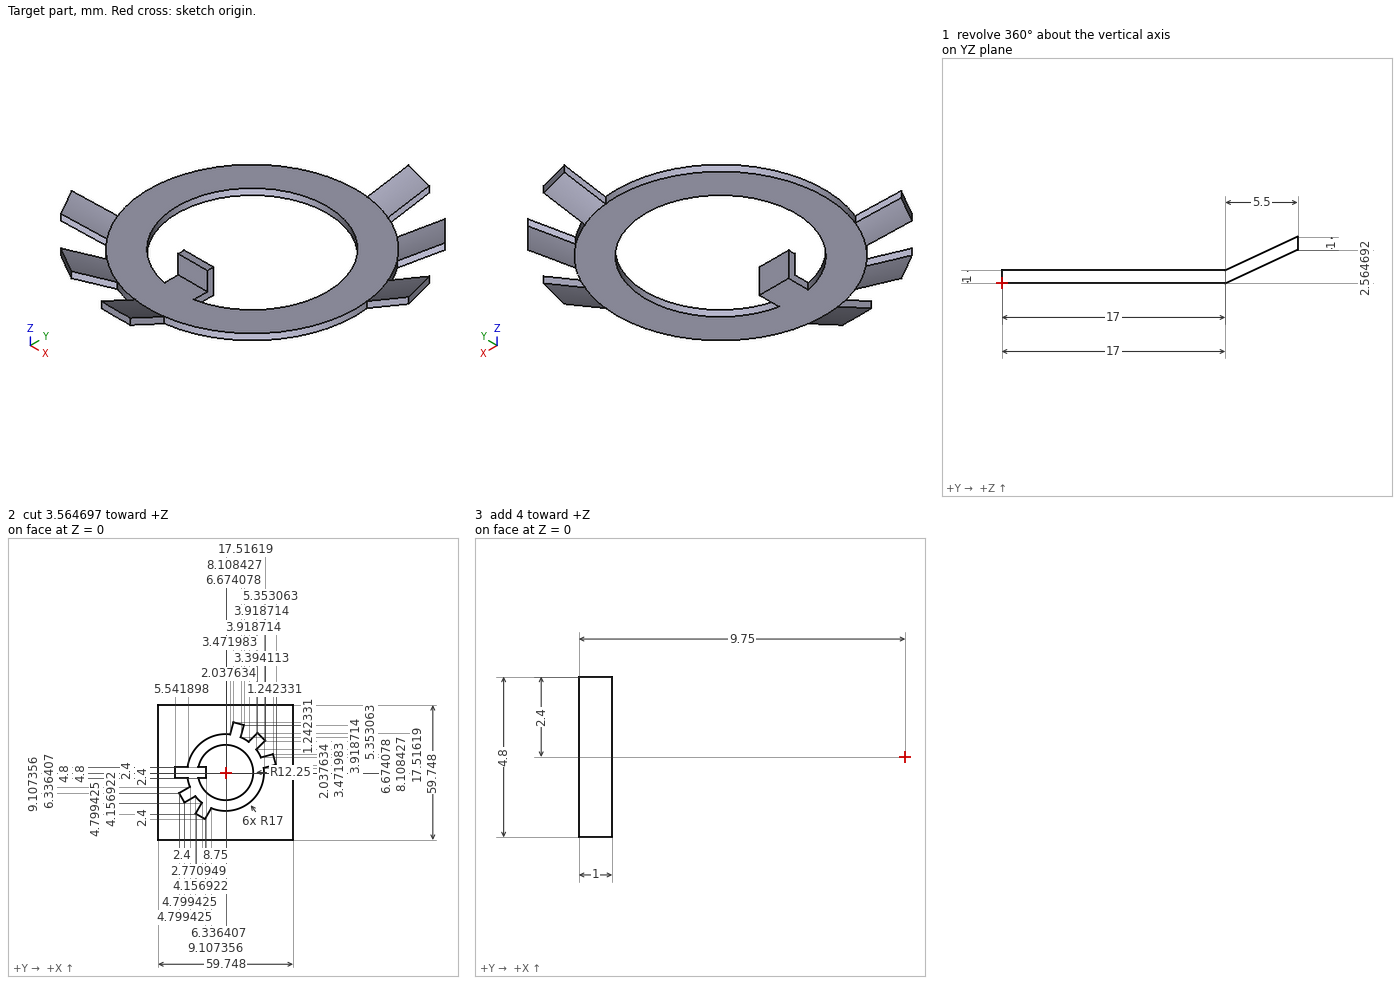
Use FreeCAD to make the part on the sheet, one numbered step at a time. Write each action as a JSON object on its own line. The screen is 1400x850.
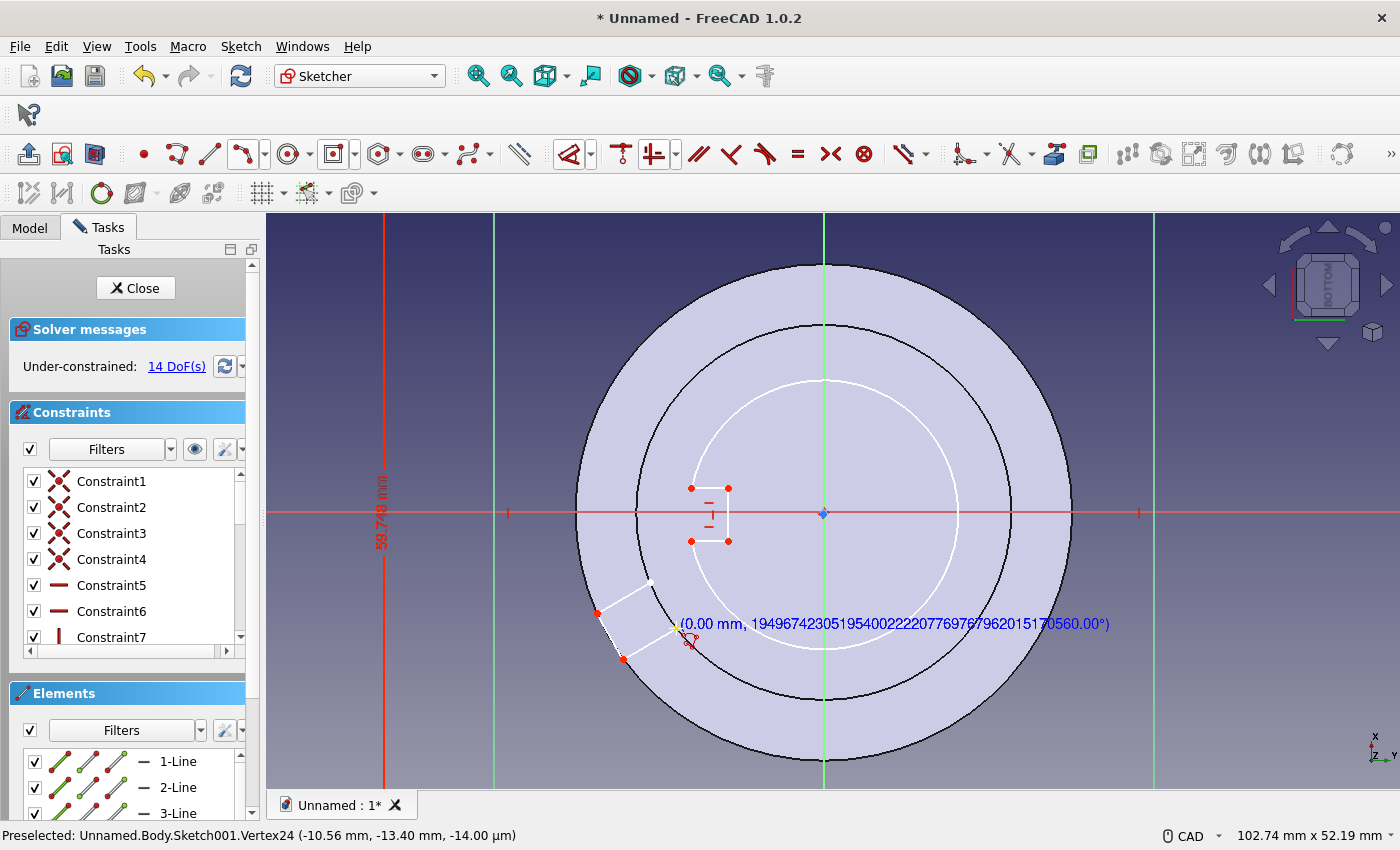
{"action": "left_click", "coordinate": [708, 660]}
{"action": "left_click", "coordinate": [677, 713]}
{"action": "left_click", "coordinate": [723, 740]}
{"action": "left_click", "coordinate": [754, 687]}
{"action": "right_click", "coordinate": [754, 687]}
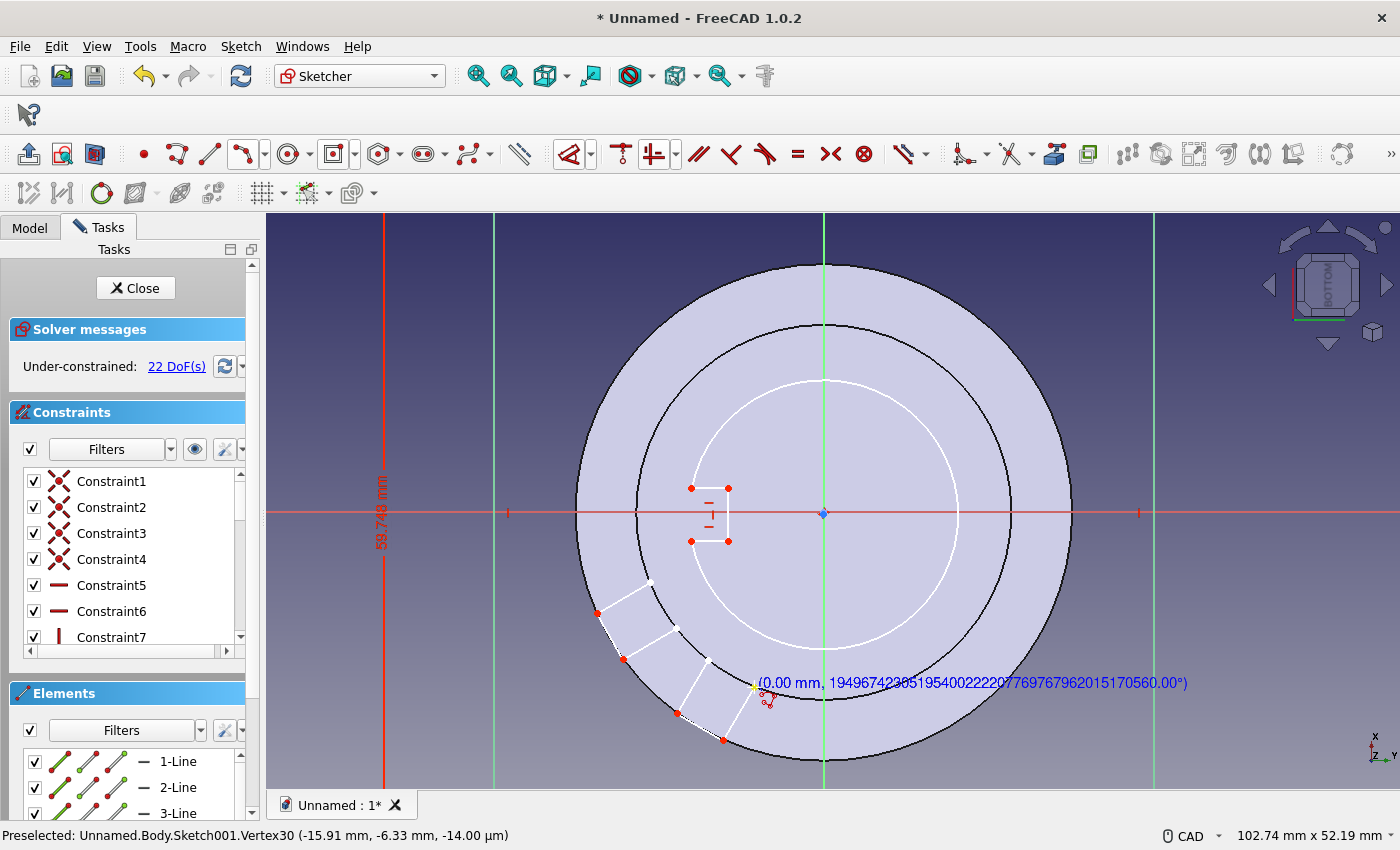
{"action": "left_click", "coordinate": [1010, 490]}
{"action": "left_click", "coordinate": [1069, 474]}
{"action": "left_click", "coordinate": [1056, 423]}
{"action": "left_click", "coordinate": [996, 439]}
{"action": "right_click", "coordinate": [996, 439]}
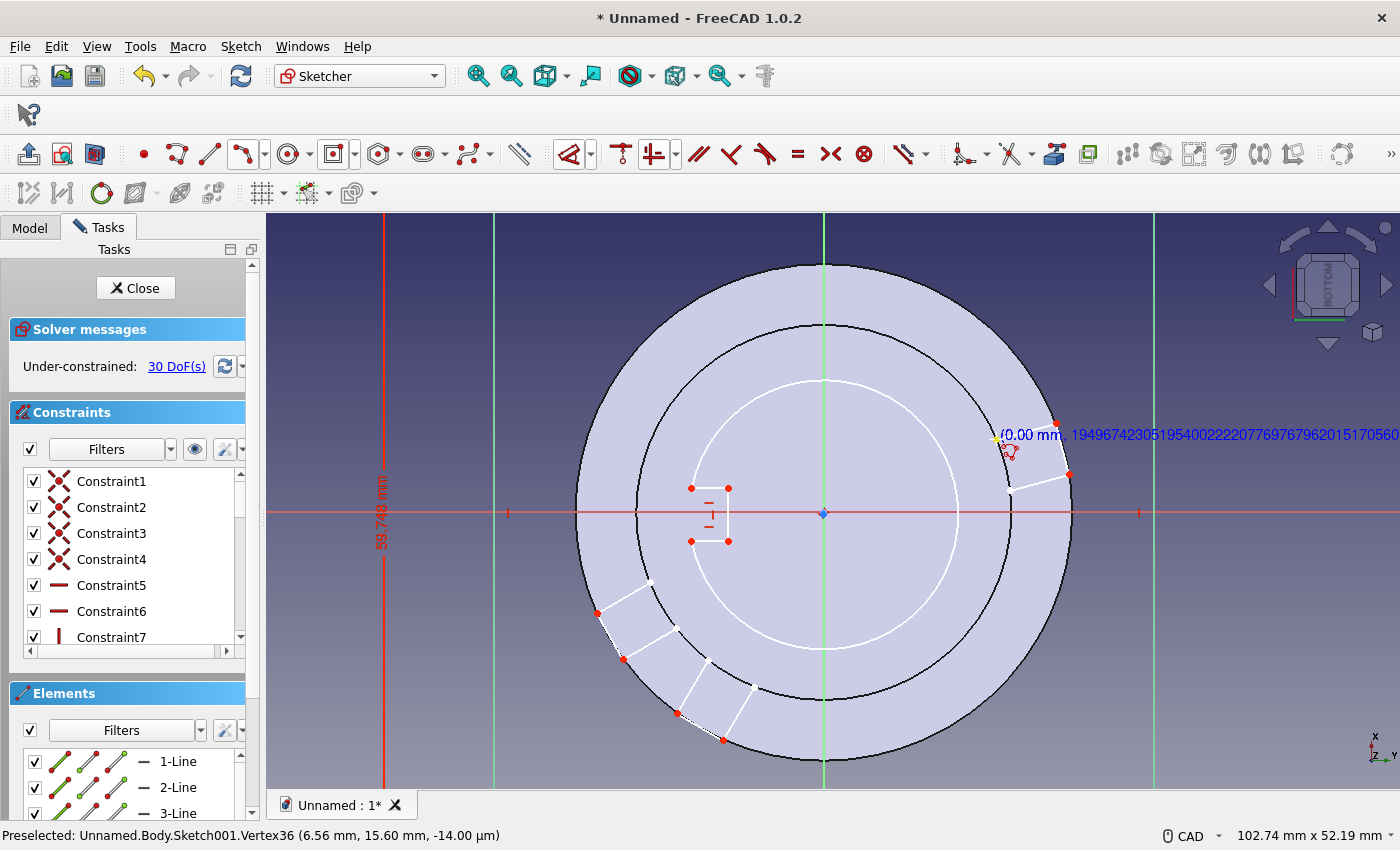
{"action": "left_click", "coordinate": [974, 400]}
{"action": "left_click", "coordinate": [1017, 357]}
{"action": "left_click", "coordinate": [980, 319]}
{"action": "left_click", "coordinate": [936, 362]}
{"action": "right_click", "coordinate": [936, 362]}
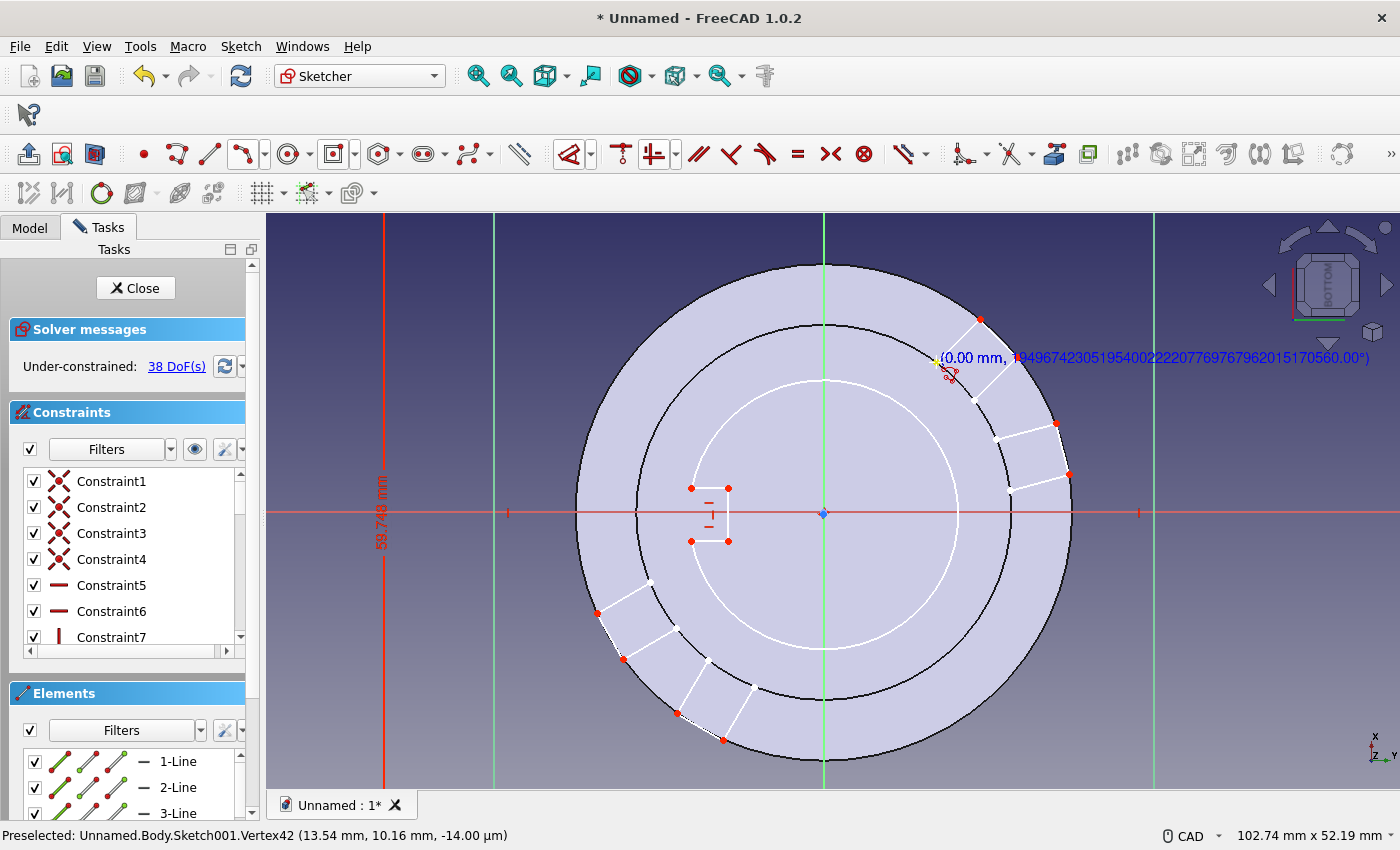
{"action": "left_click", "coordinate": [898, 340]}
{"action": "left_click", "coordinate": [913, 281]}
{"action": "left_click", "coordinate": [862, 267]}
{"action": "left_click", "coordinate": [846, 326]}
{"action": "right_click", "coordinate": [846, 326]}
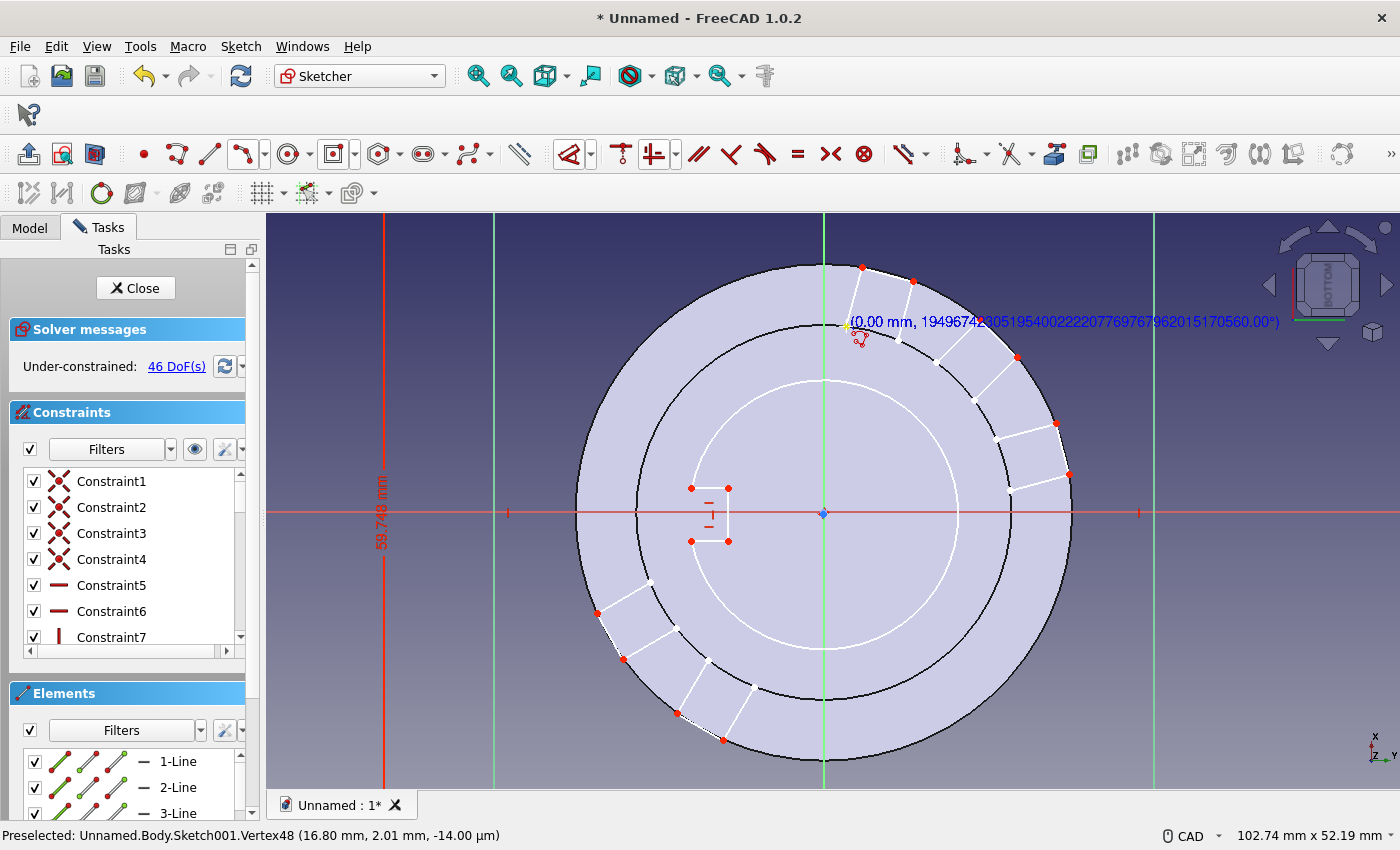
{"action": "left_click", "coordinate": [638, 486]}
{"action": "left_click", "coordinate": [577, 486]}
{"action": "left_click", "coordinate": [577, 539]}
{"action": "left_click", "coordinate": [638, 539]}
{"action": "right_click", "coordinate": [638, 539]}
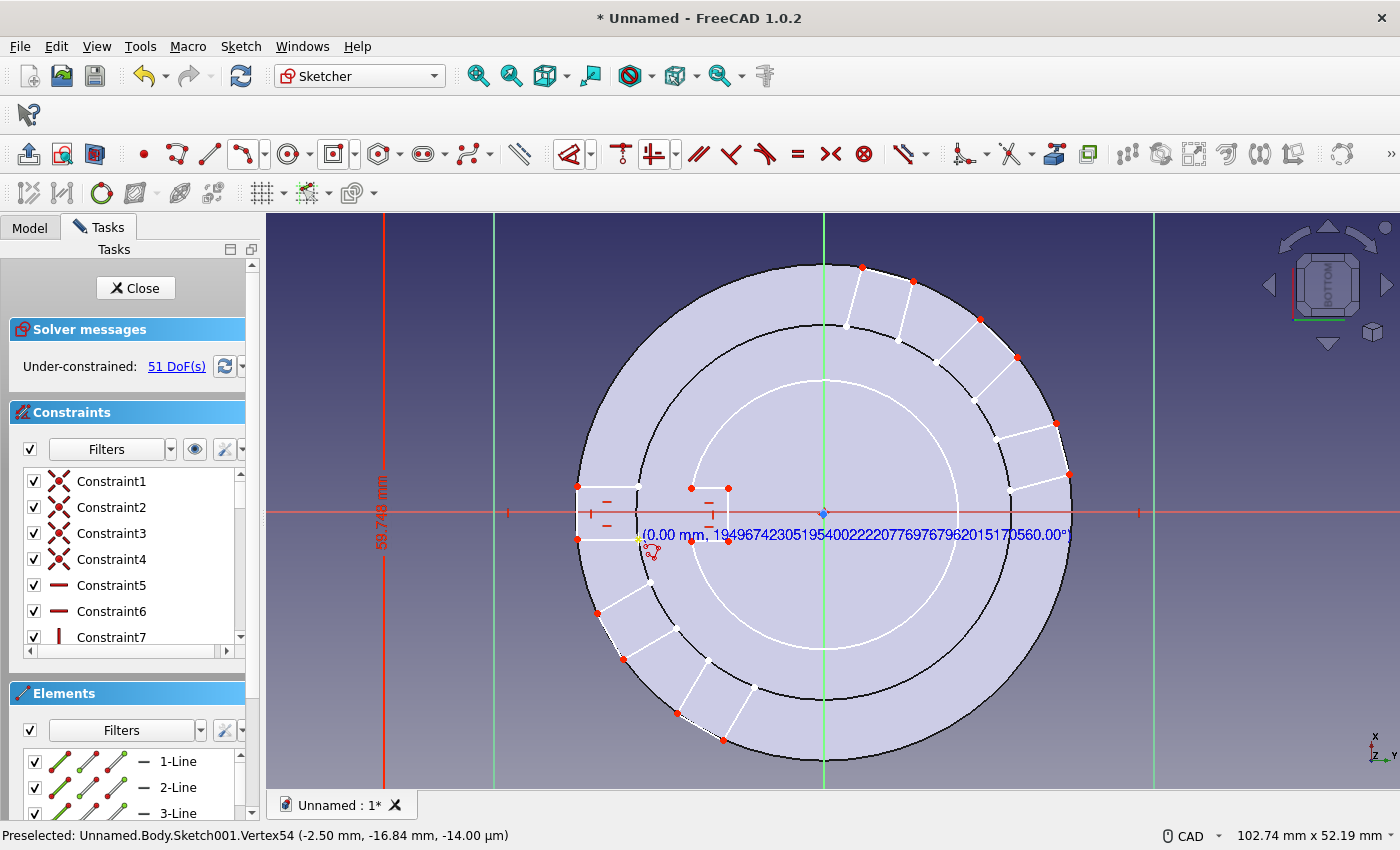
{"action": "left_click", "coordinate": [242, 154]}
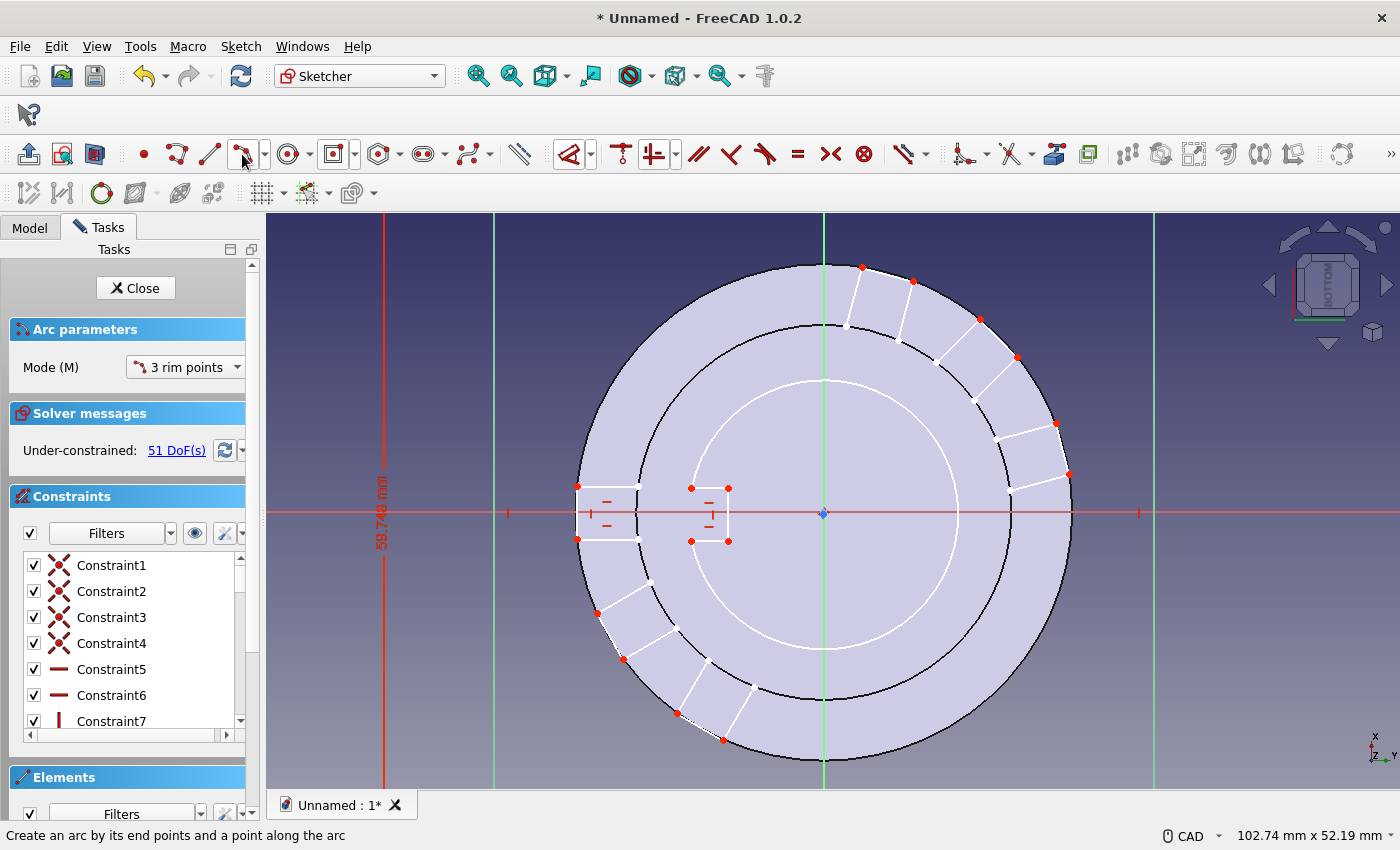
{"action": "left_click", "coordinate": [676, 629]}
{"action": "left_click", "coordinate": [708, 661]}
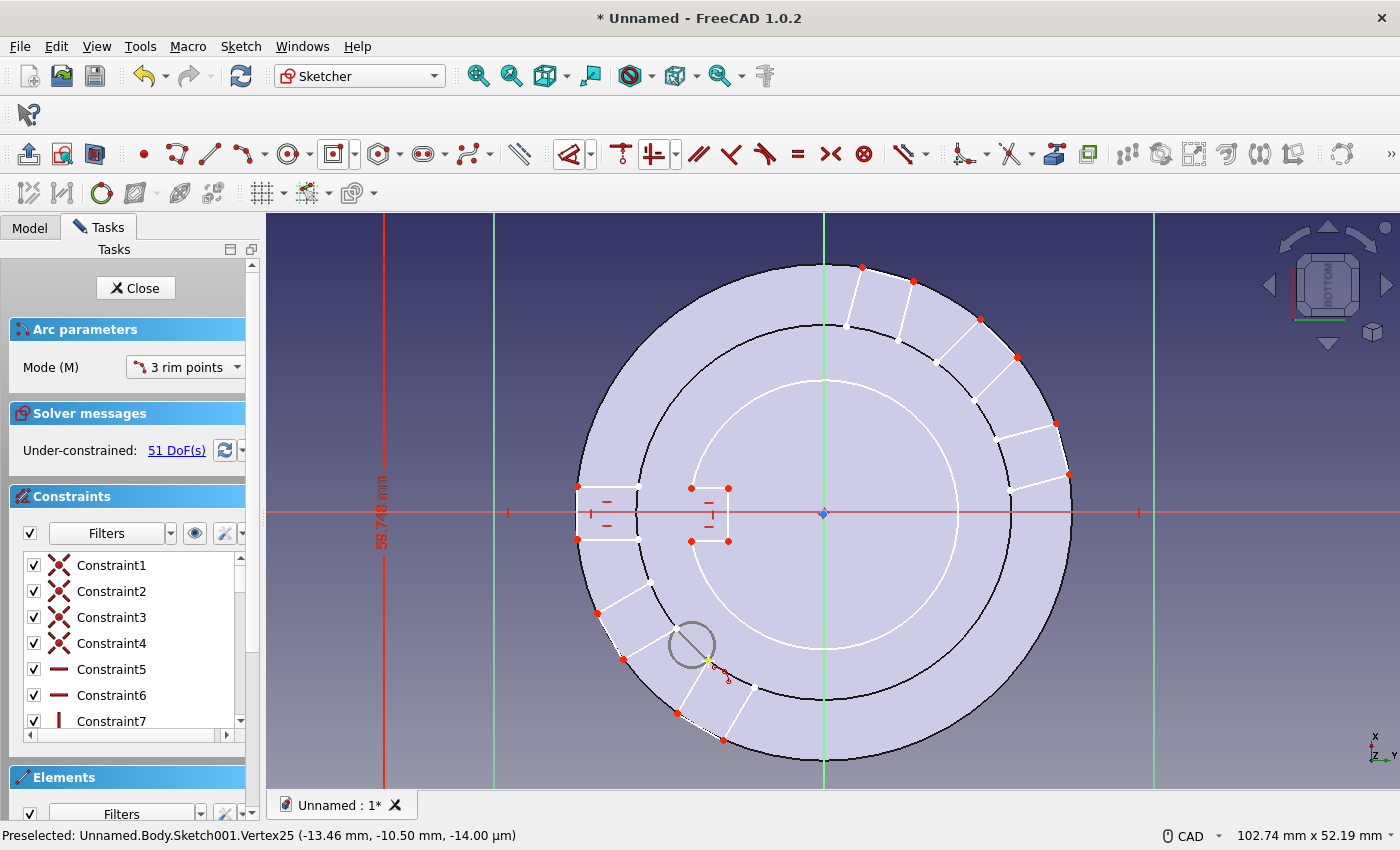
{"action": "scroll", "coordinate": [691, 645], "scroll_direction": "up", "scroll_amount": 13}